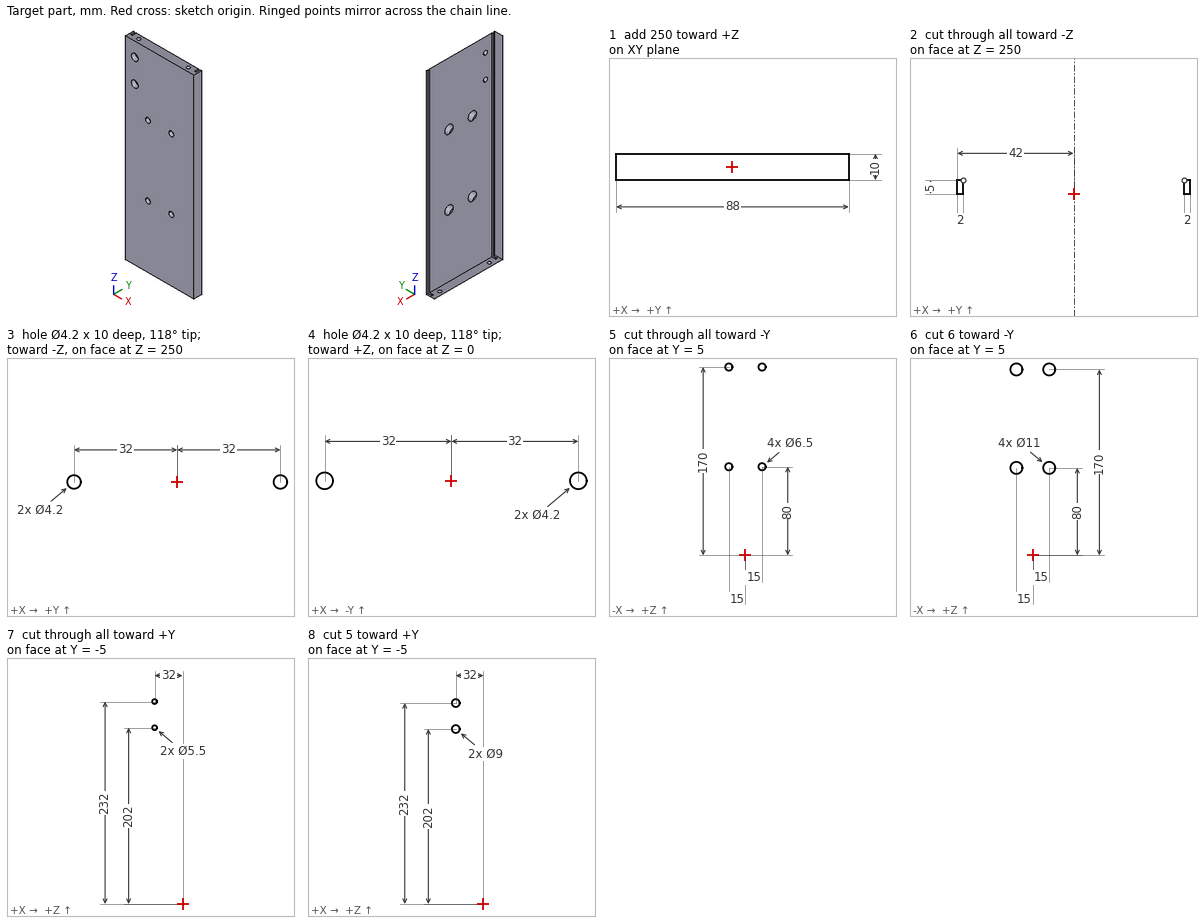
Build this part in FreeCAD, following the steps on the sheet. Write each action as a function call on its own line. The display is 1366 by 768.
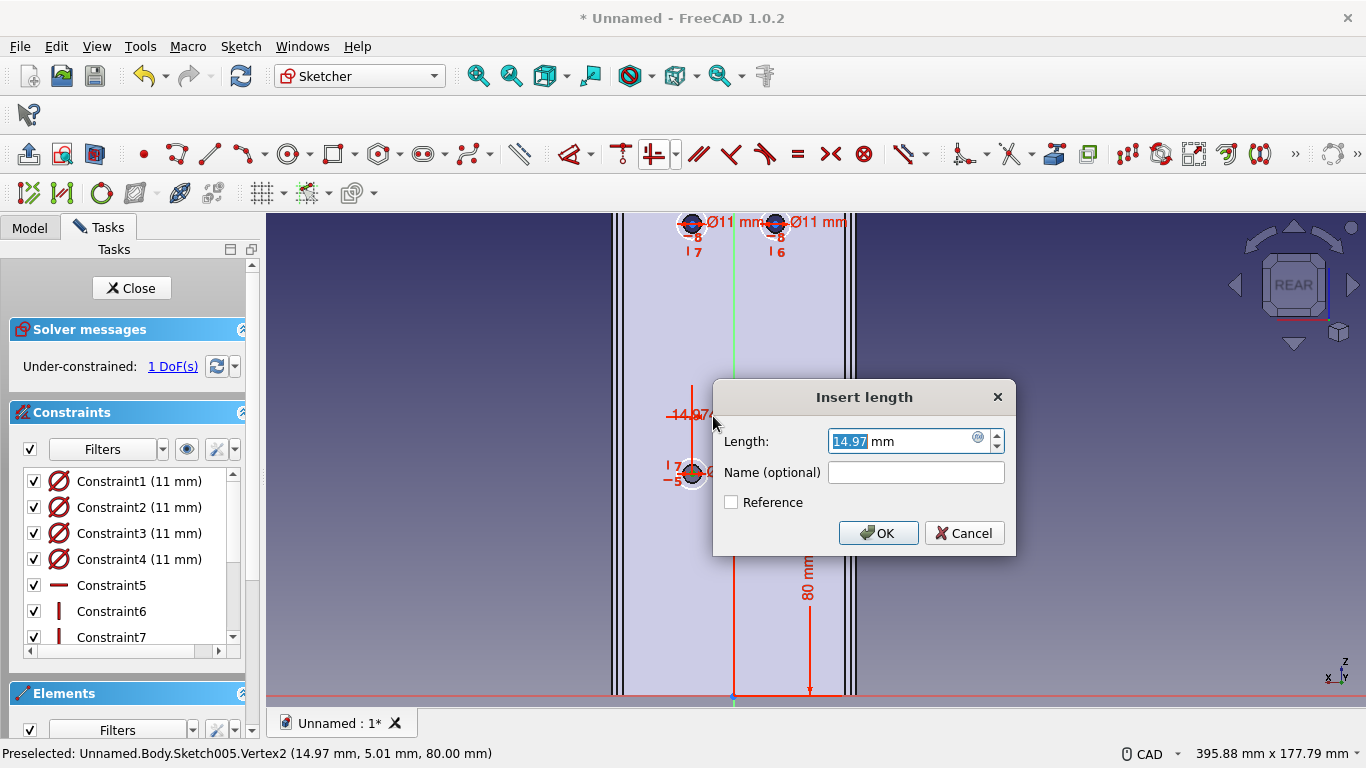
text(15)
key(Return)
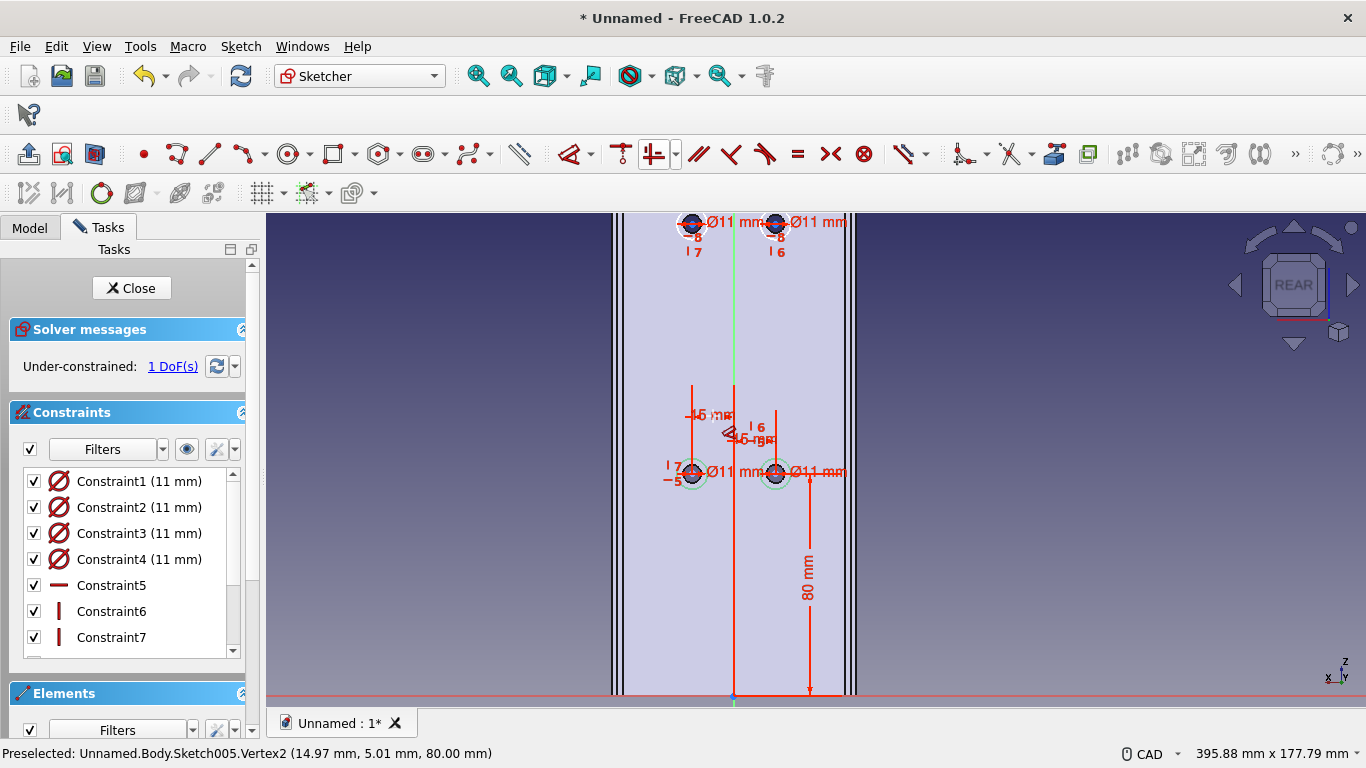
scroll(775, 475, down, 2)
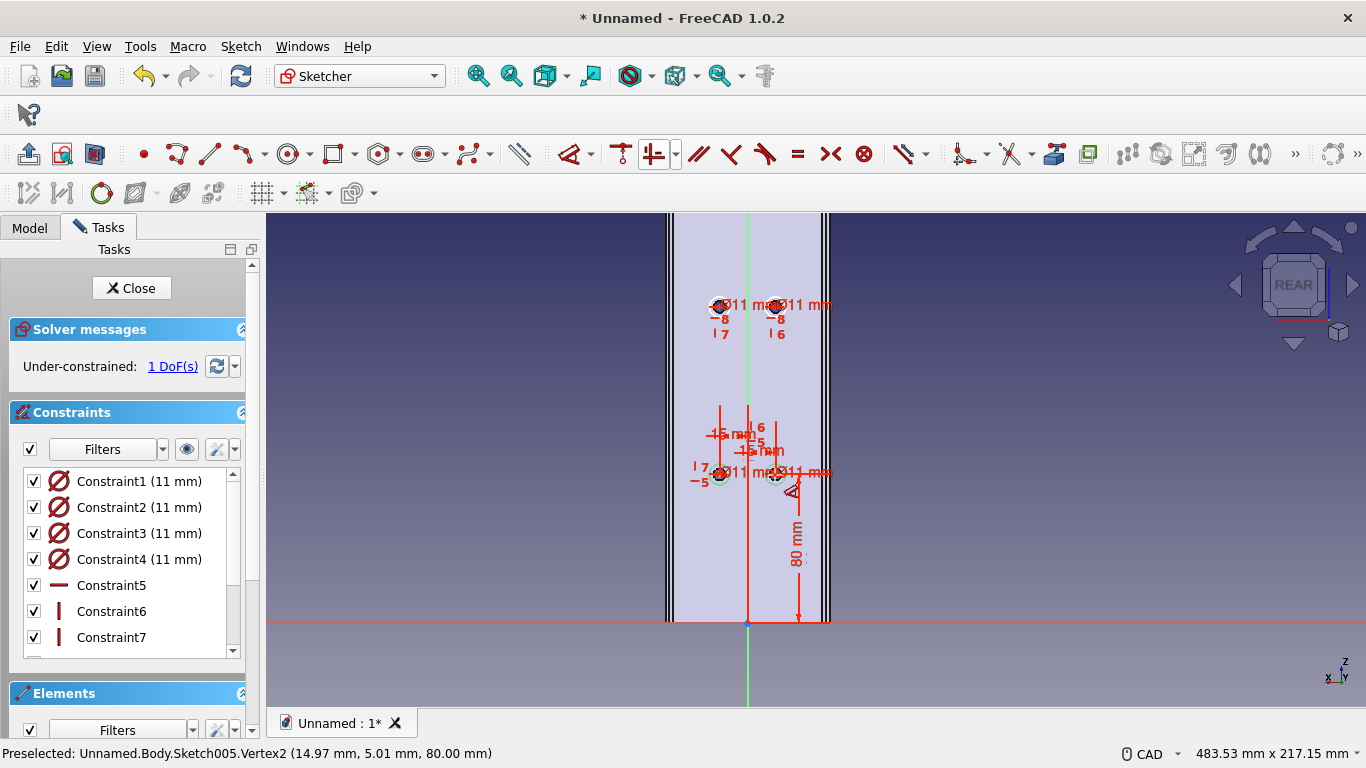
click(776, 307)
click(810, 393)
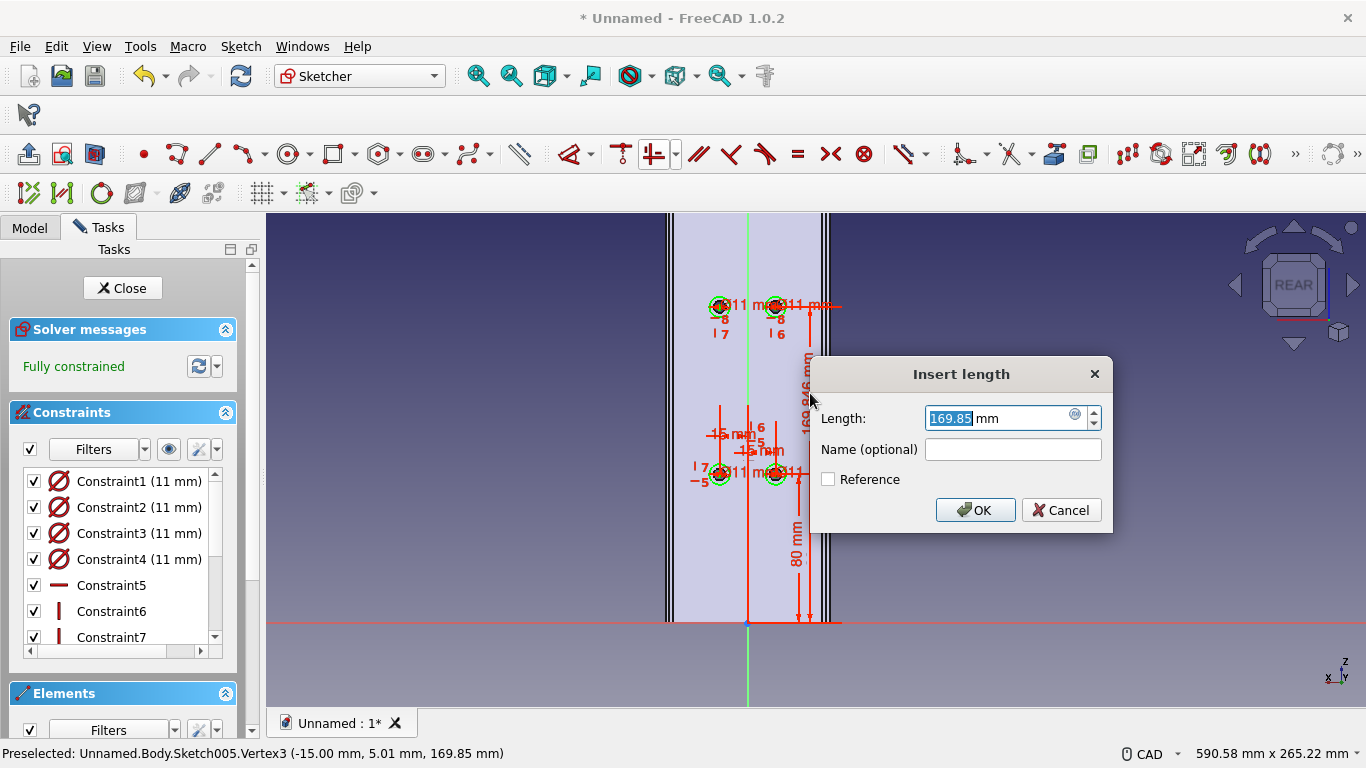
text(170)
key(Return)
key(Escape)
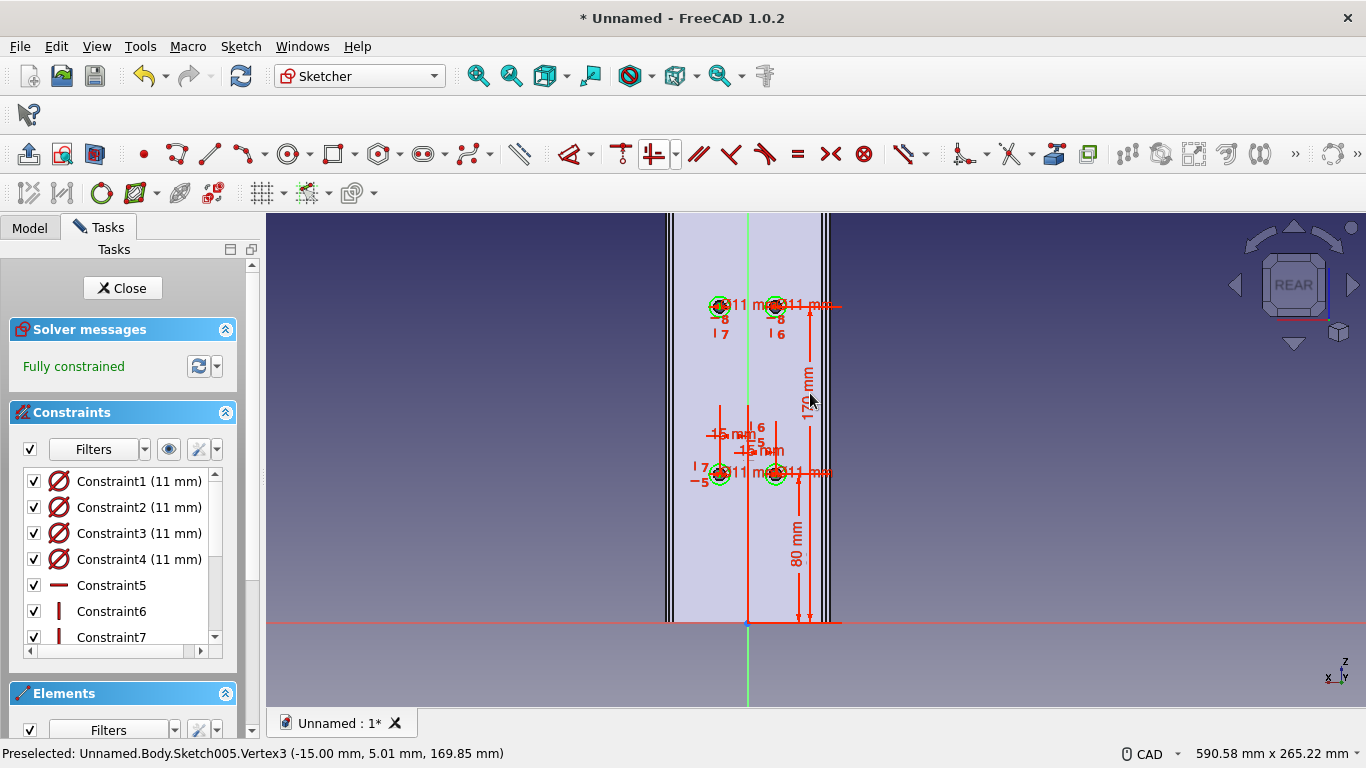
click(123, 288)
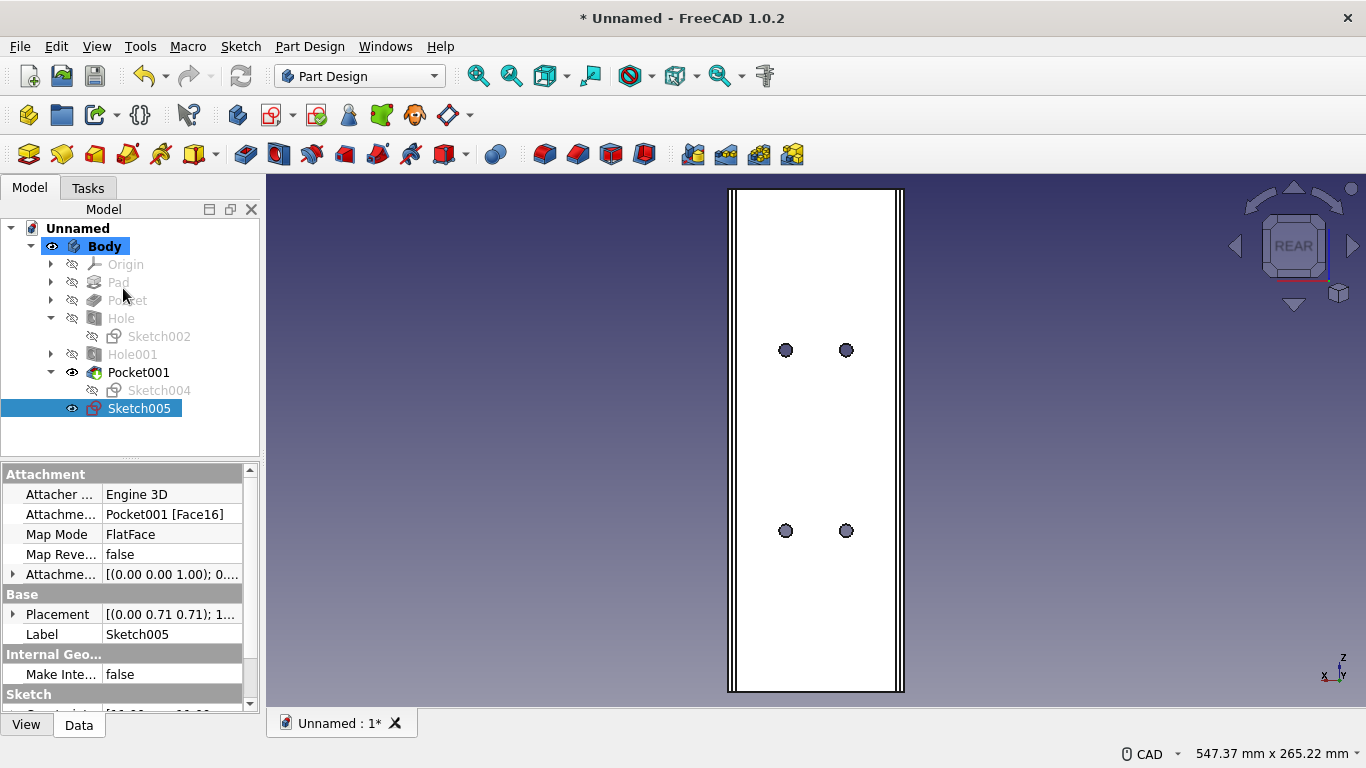
click(246, 154)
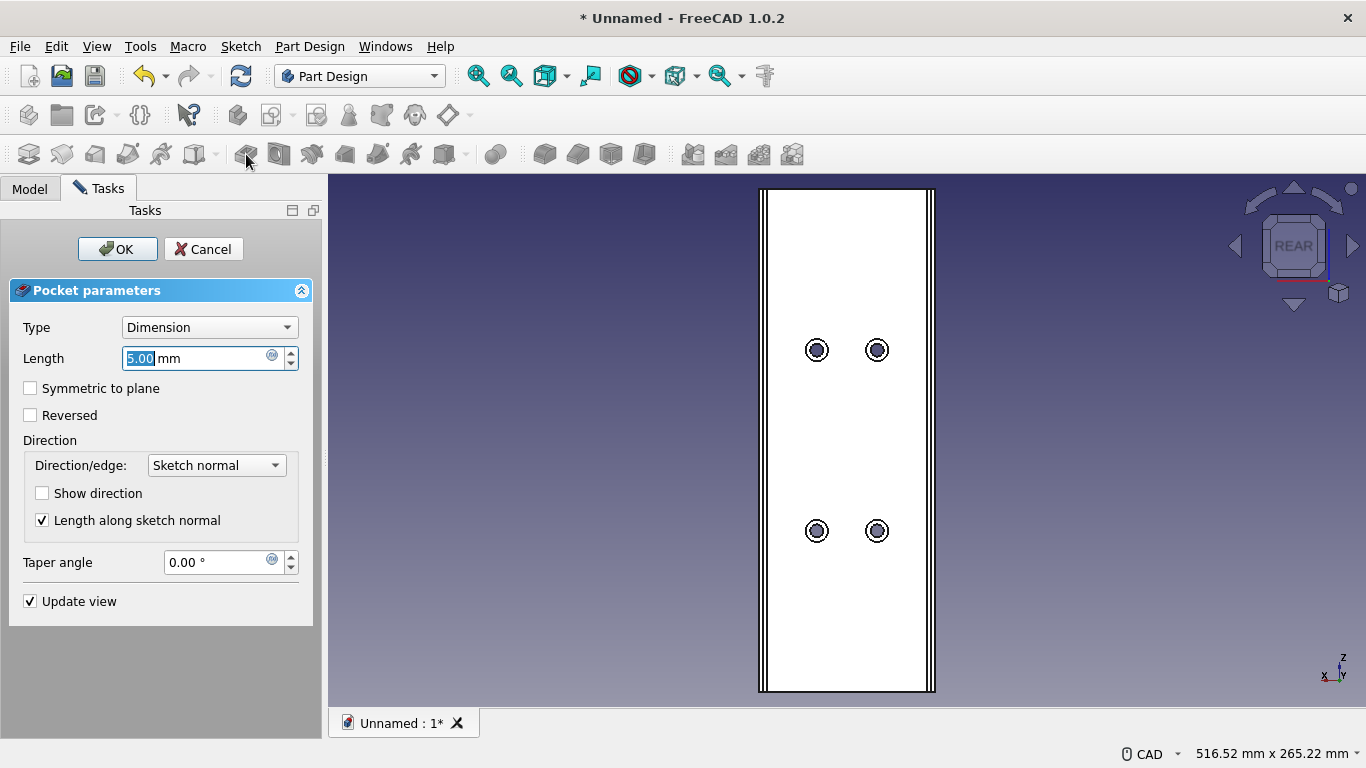
text(6)
key(Tab)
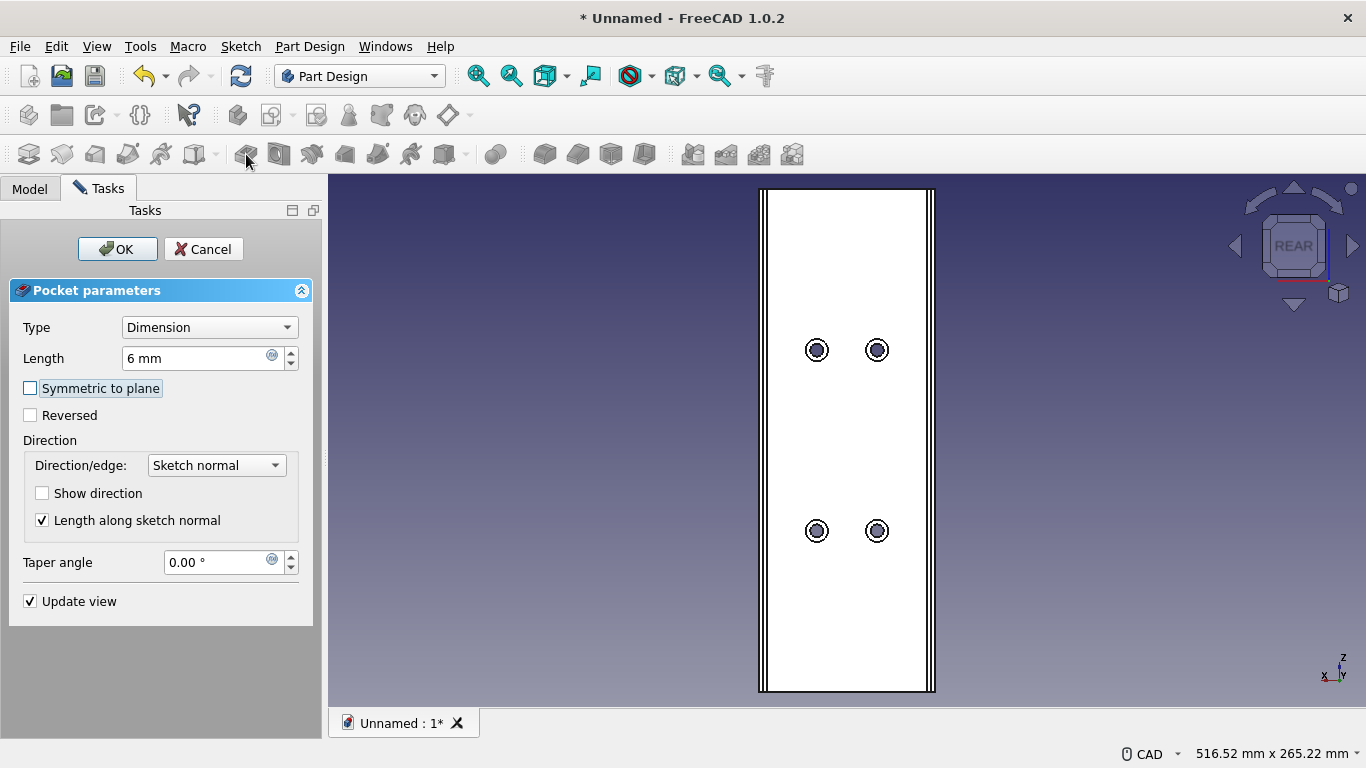
click(118, 249)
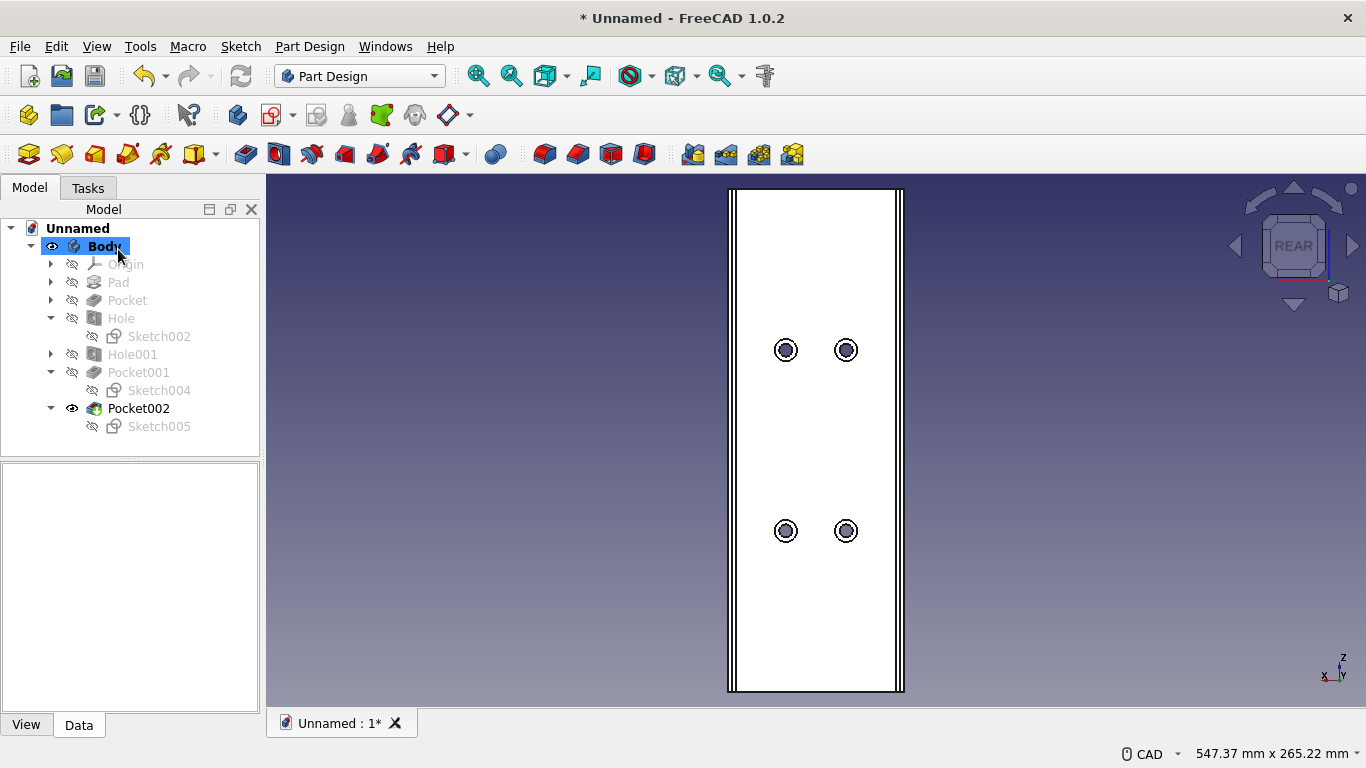
key(0)